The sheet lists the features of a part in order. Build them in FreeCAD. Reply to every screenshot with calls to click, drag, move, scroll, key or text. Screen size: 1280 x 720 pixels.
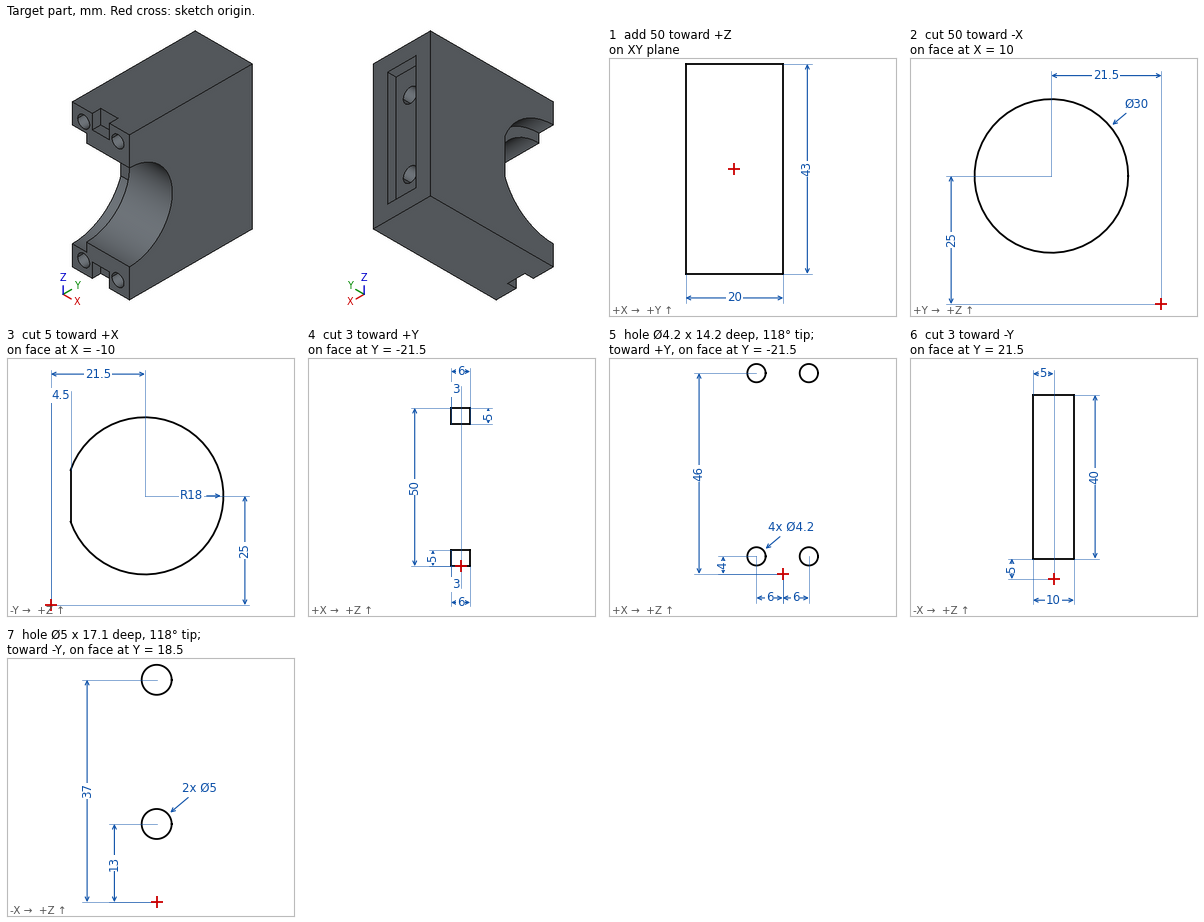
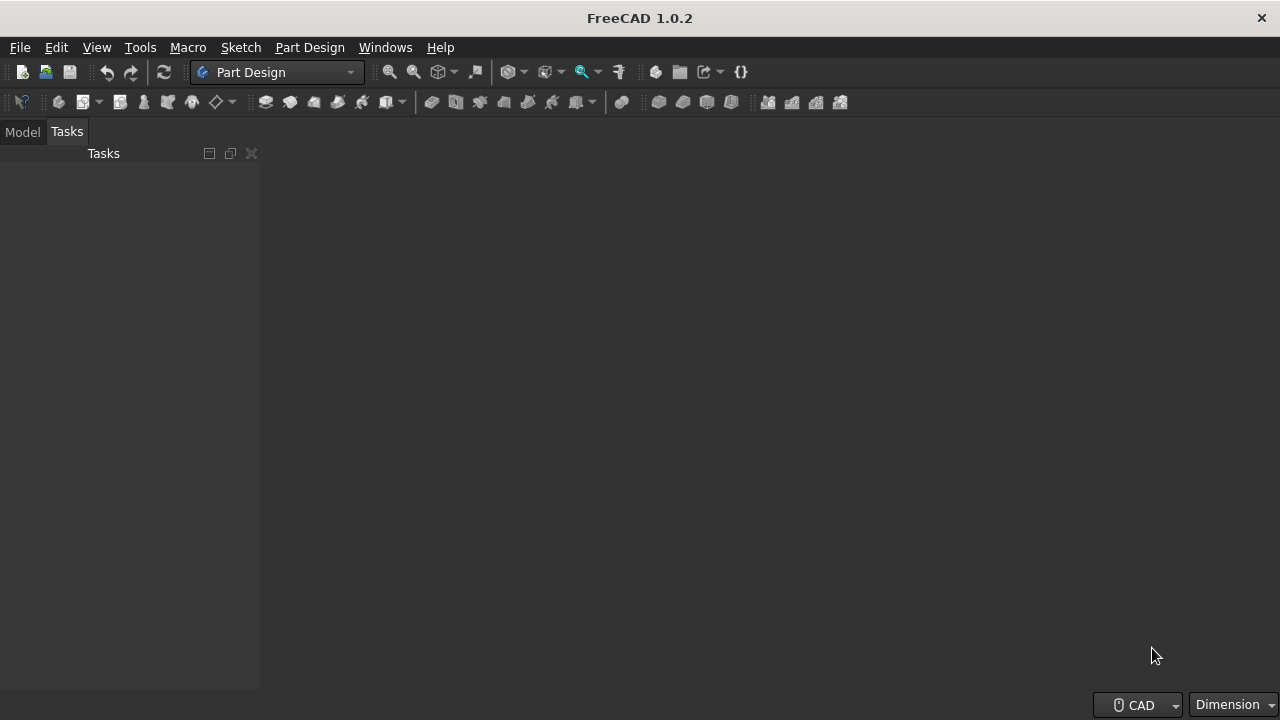
click(22, 72)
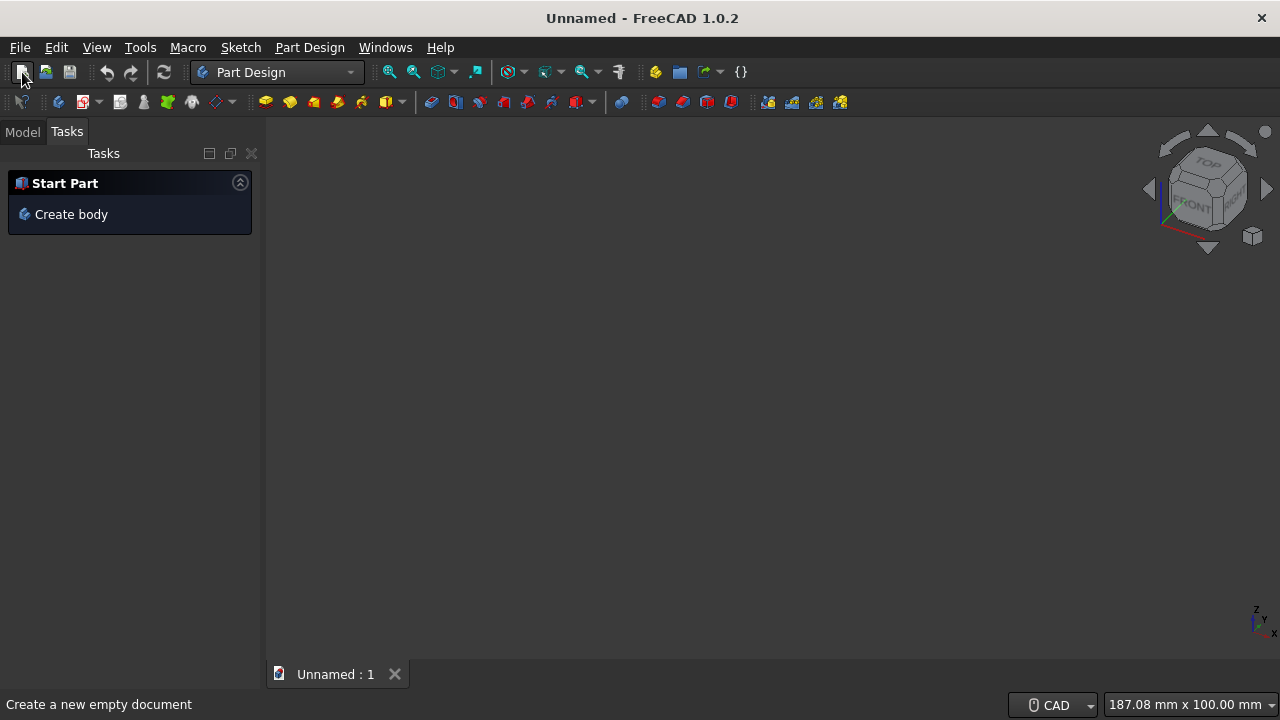
click(84, 102)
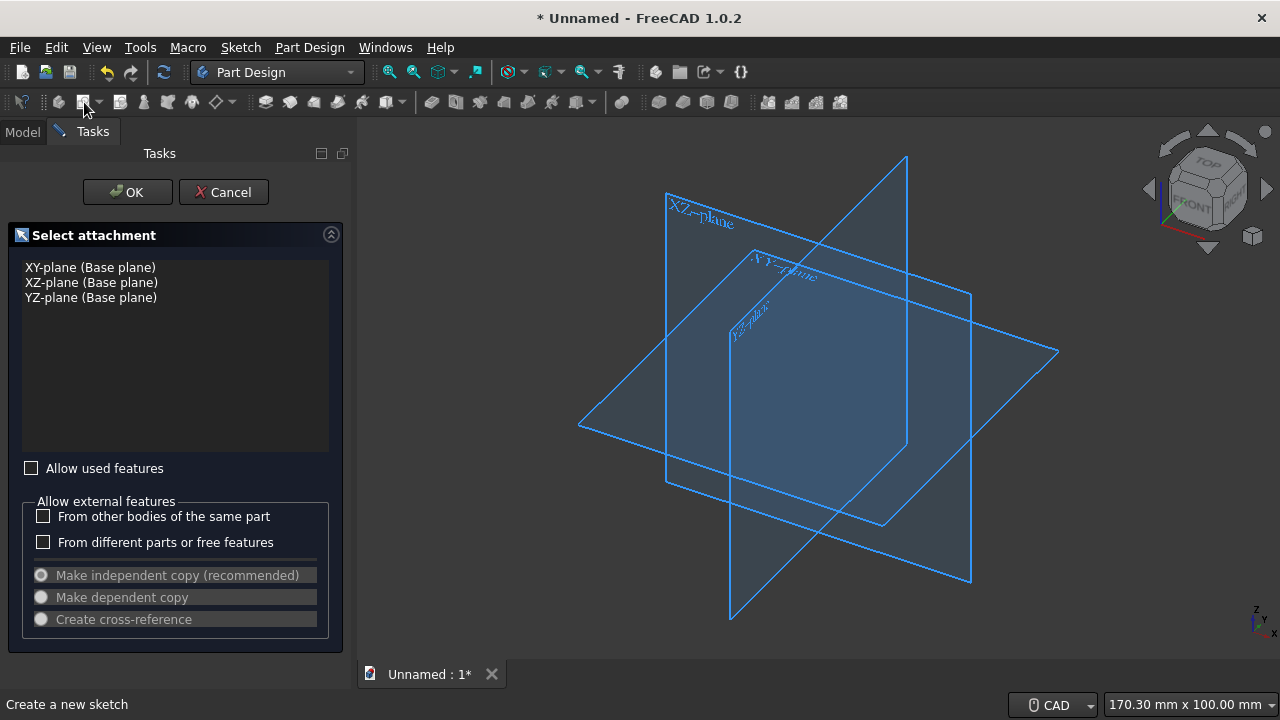
click(82, 268)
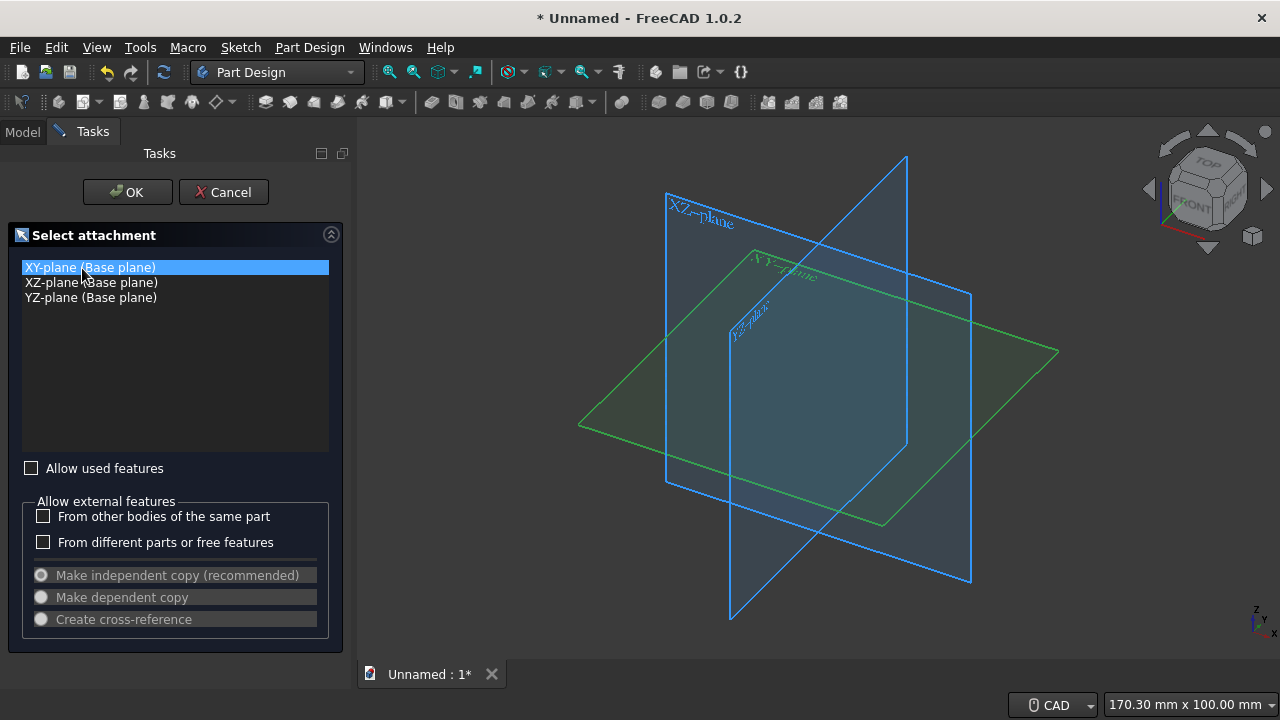
click(128, 192)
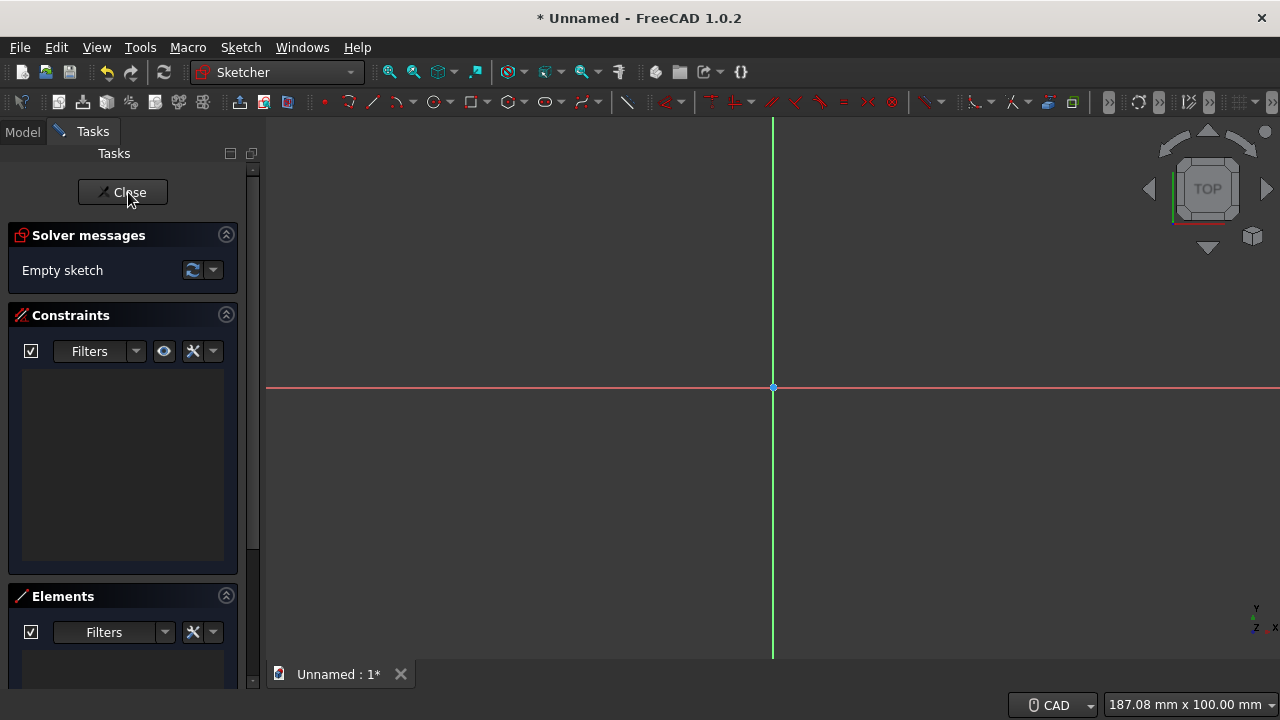
scroll(912, 388, up, 2)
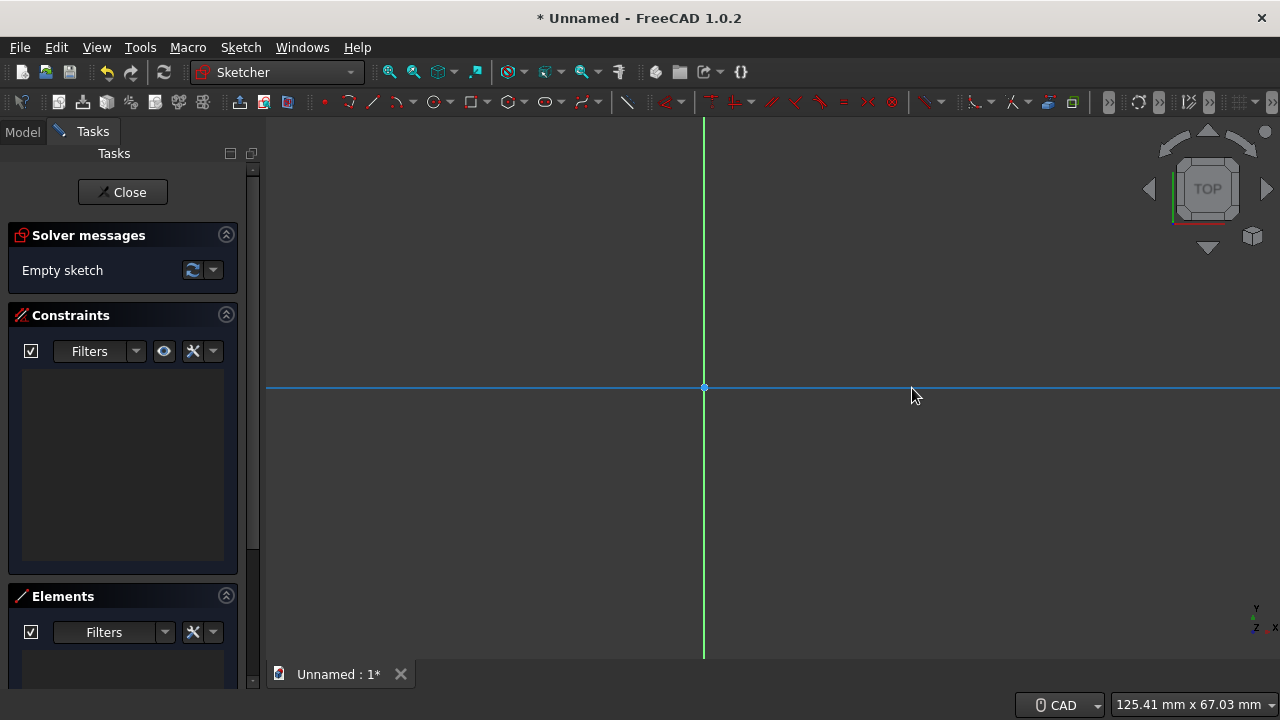
click(490, 102)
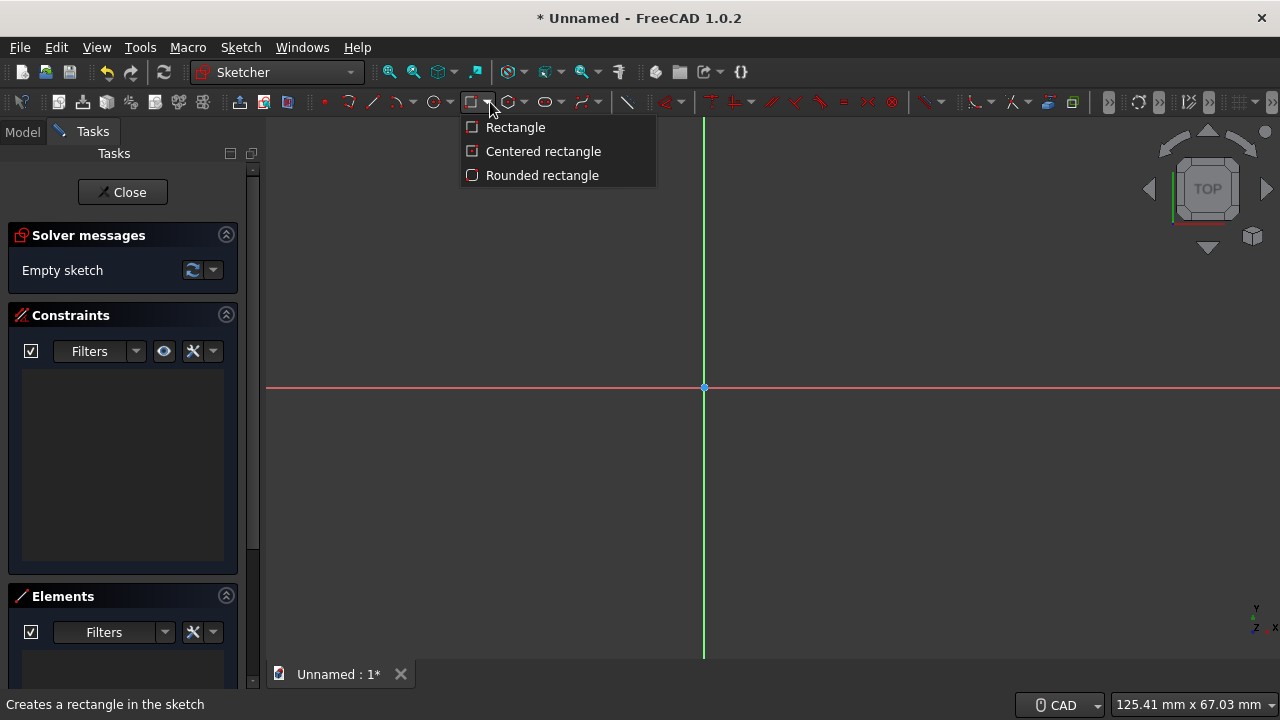
click(558, 151)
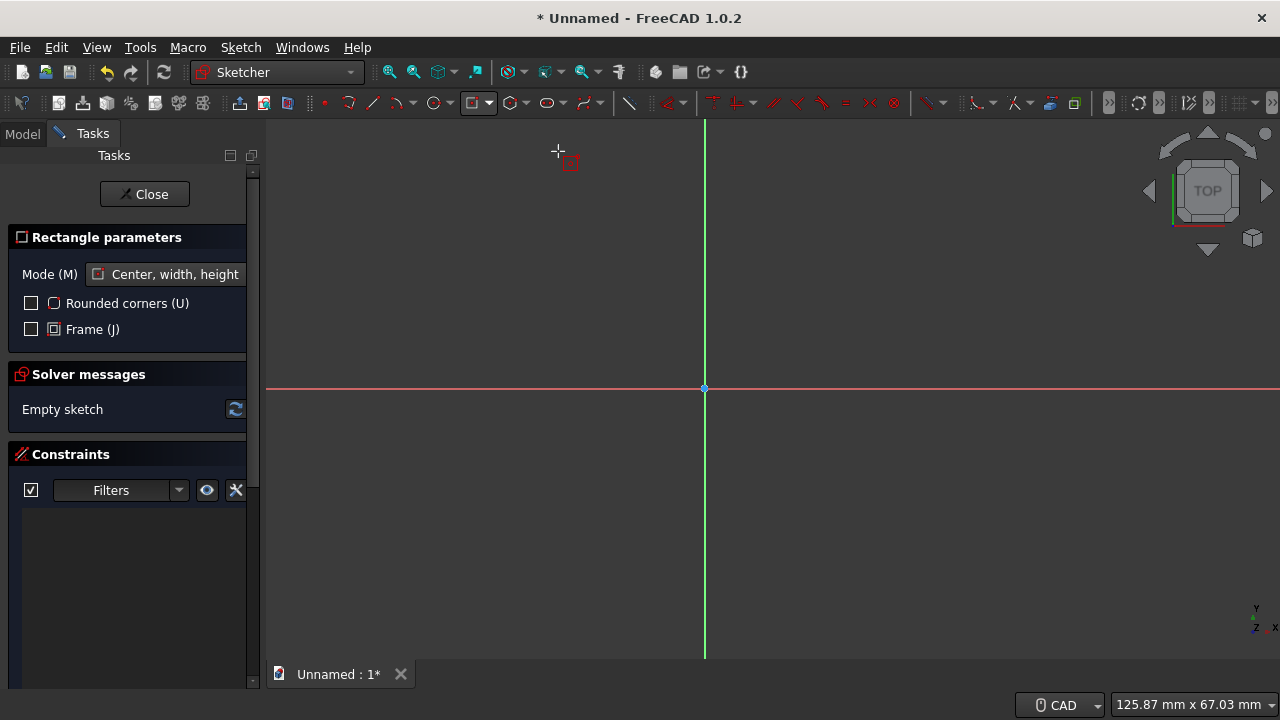
click(705, 389)
move(785, 216)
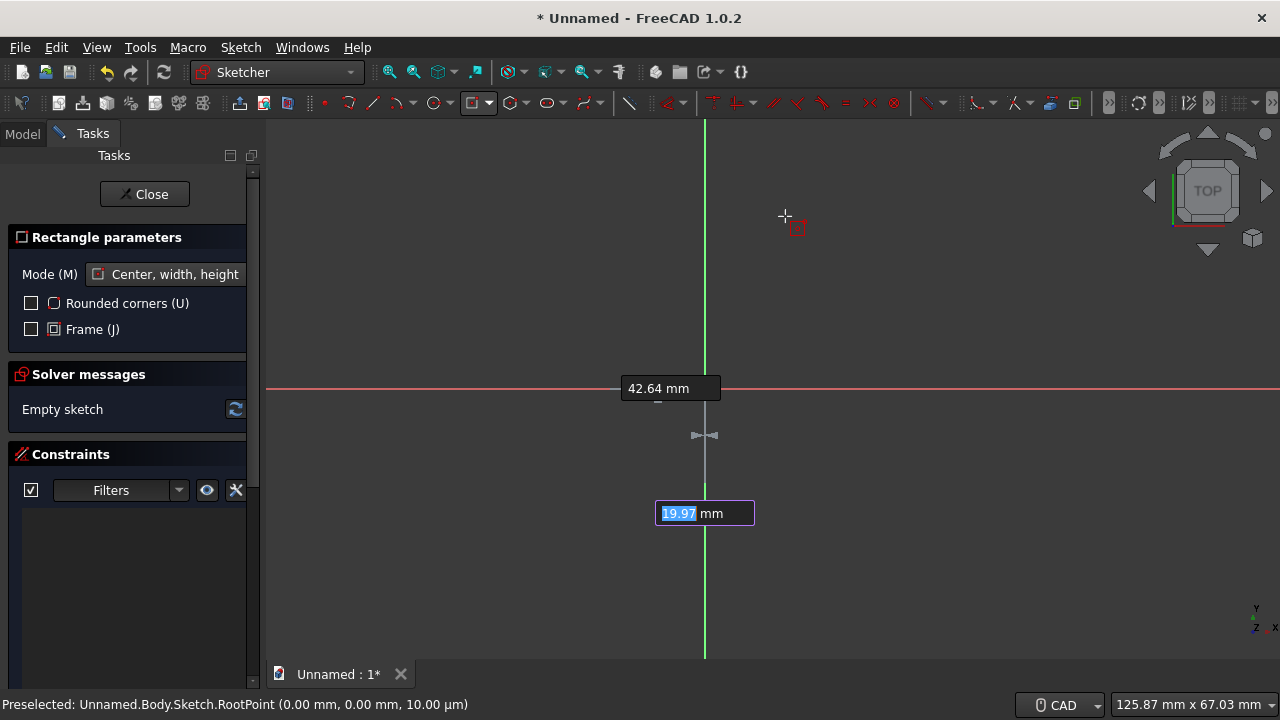
text(20)
key(Tab)
text(43)
key(Return)
key(Escape)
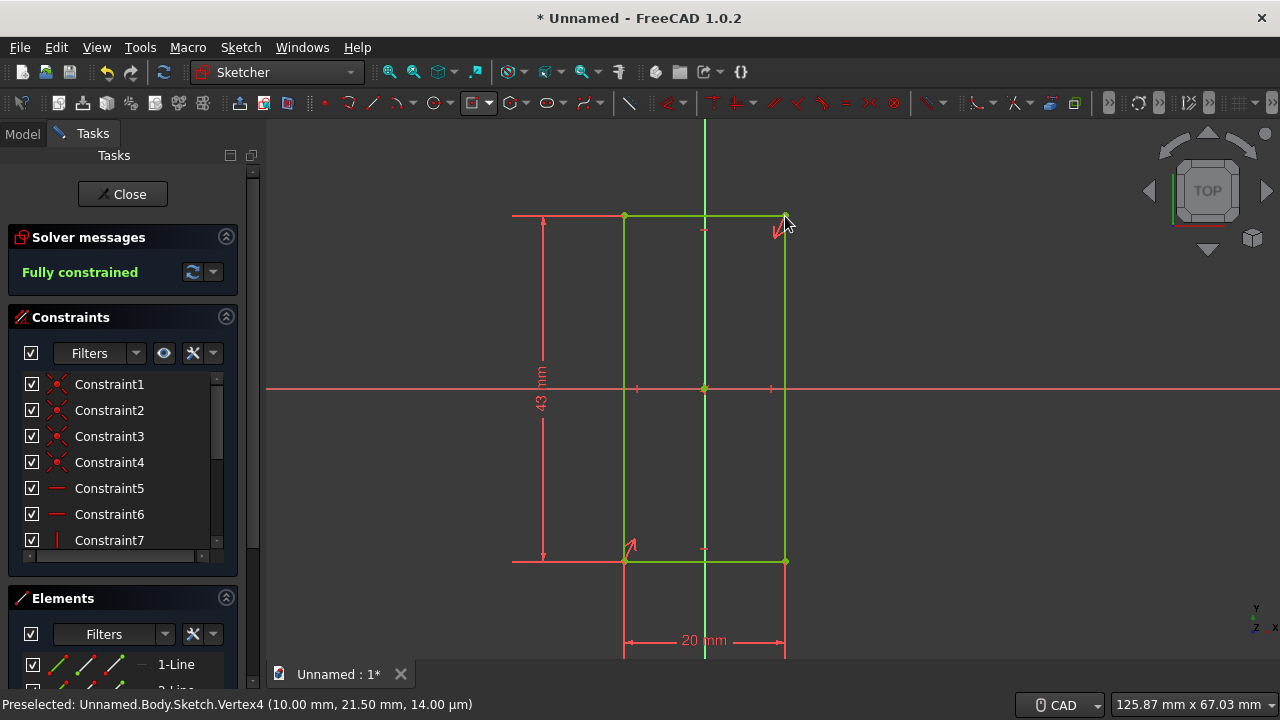
click(123, 194)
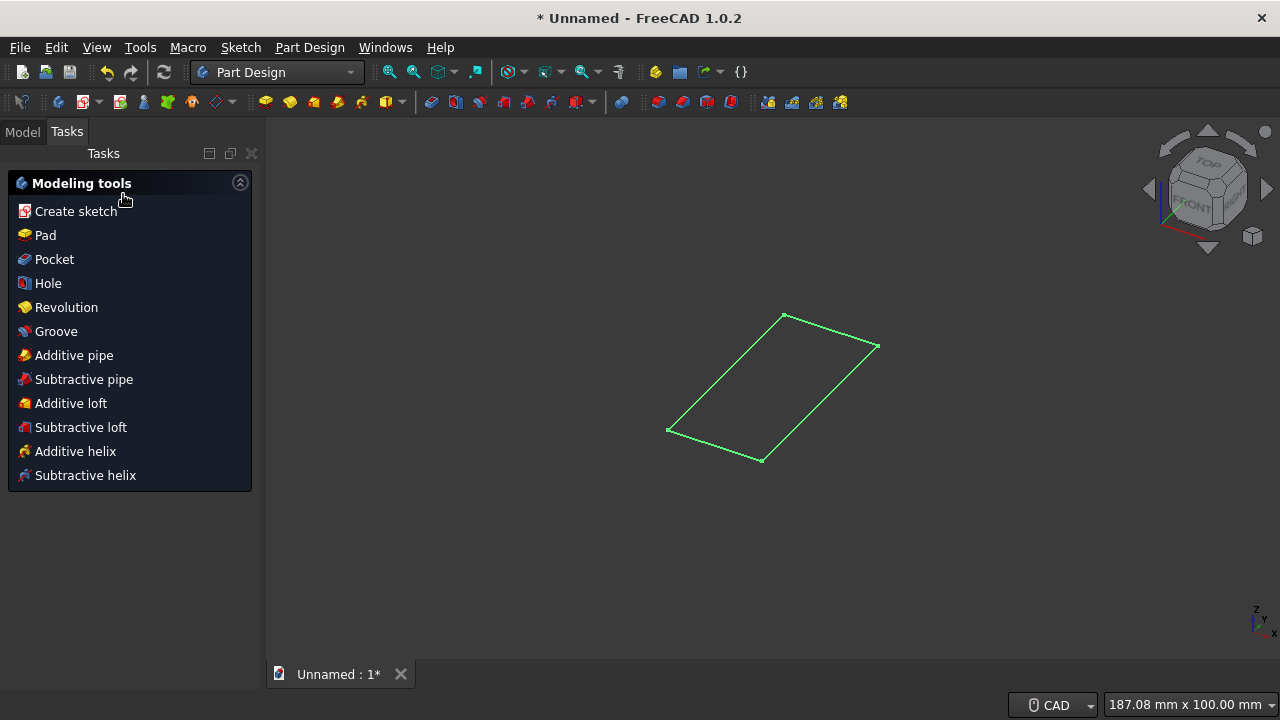
click(266, 102)